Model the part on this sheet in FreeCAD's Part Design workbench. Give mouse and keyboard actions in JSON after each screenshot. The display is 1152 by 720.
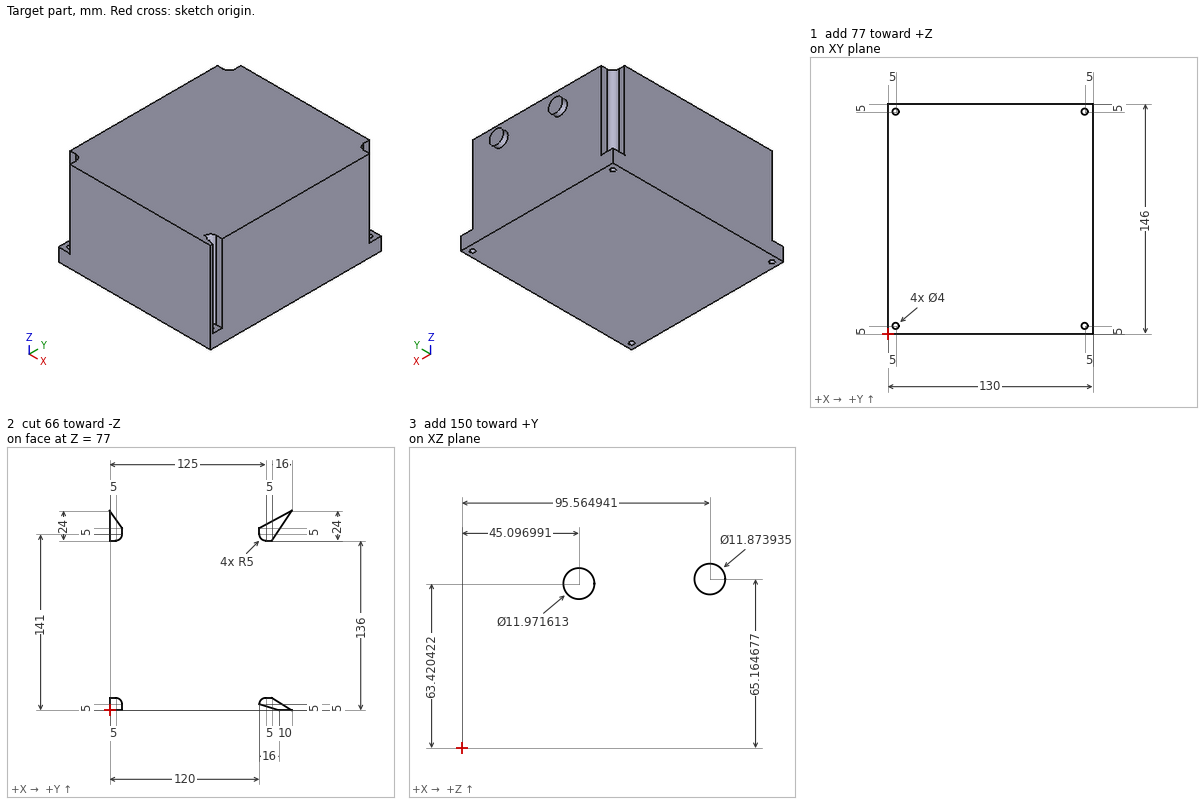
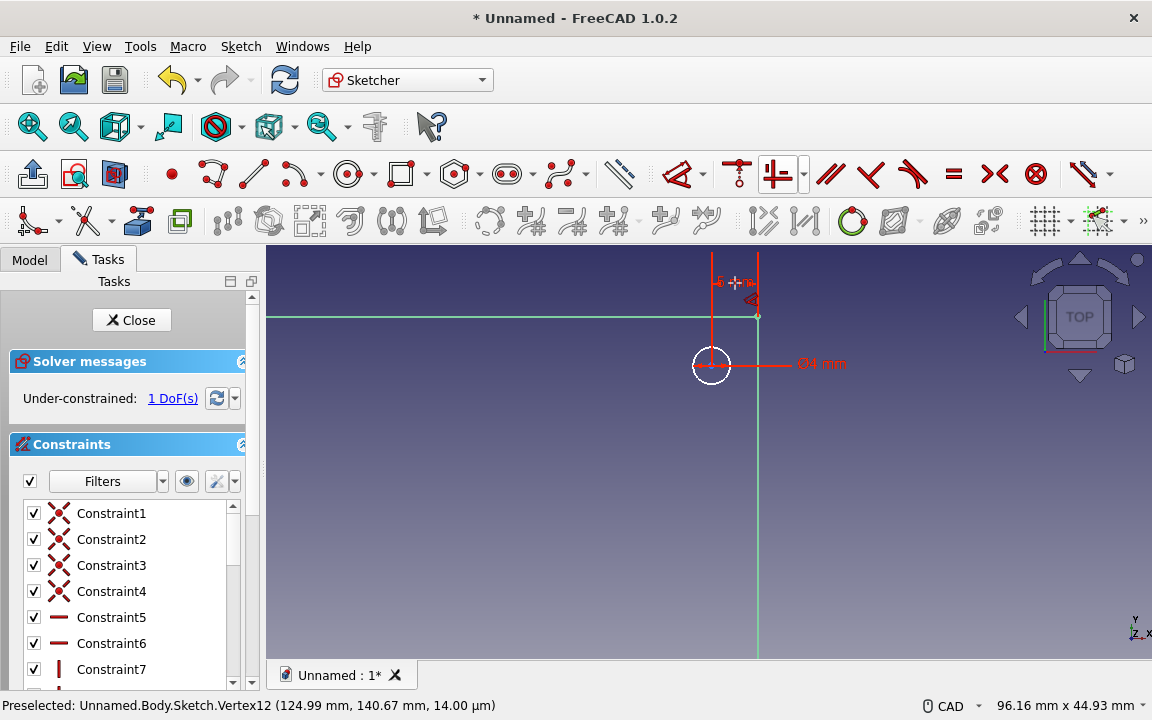
{"action": "left_click", "coordinate": [758, 317]}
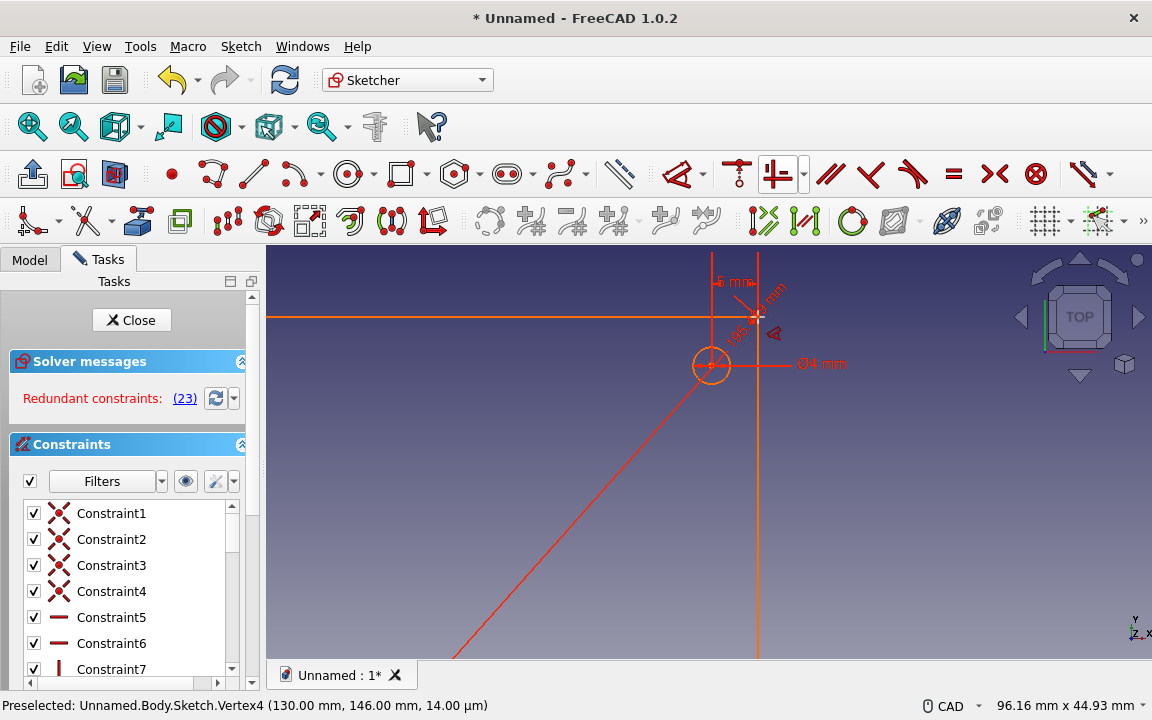
{"action": "left_click", "coordinate": [712, 366]}
{"action": "left_click", "coordinate": [792, 341]}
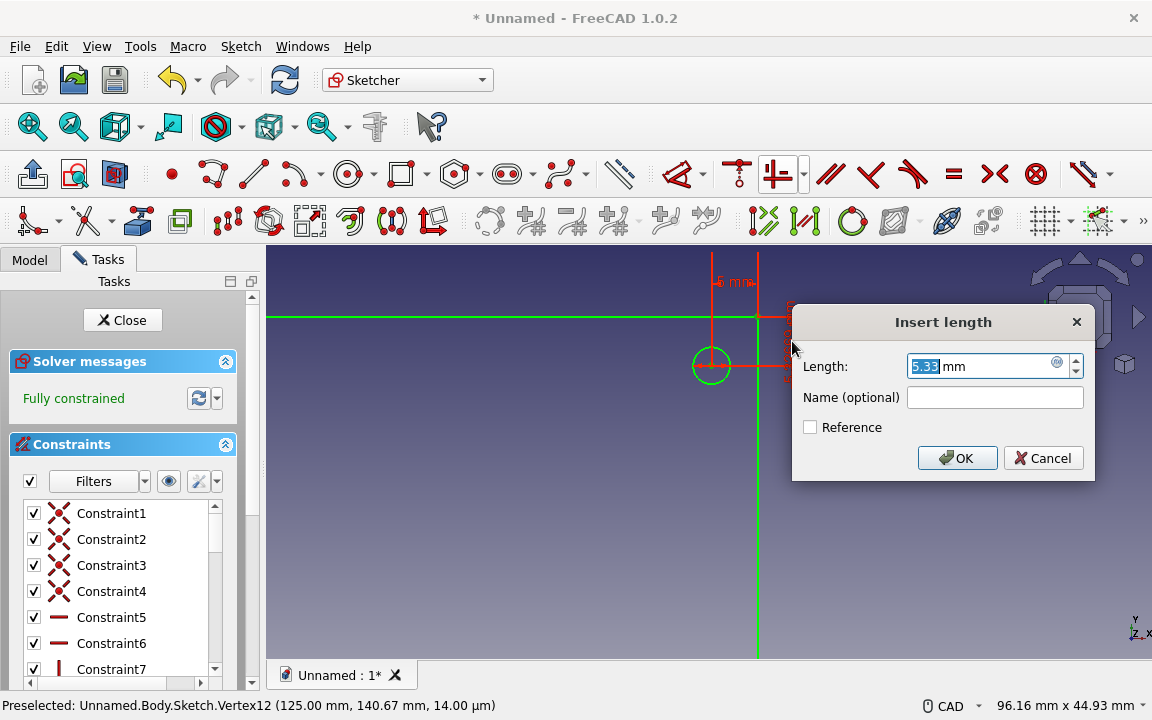
{"action": "type", "text": "5"}
{"action": "key", "text": "Return"}
{"action": "key", "text": "Escape"}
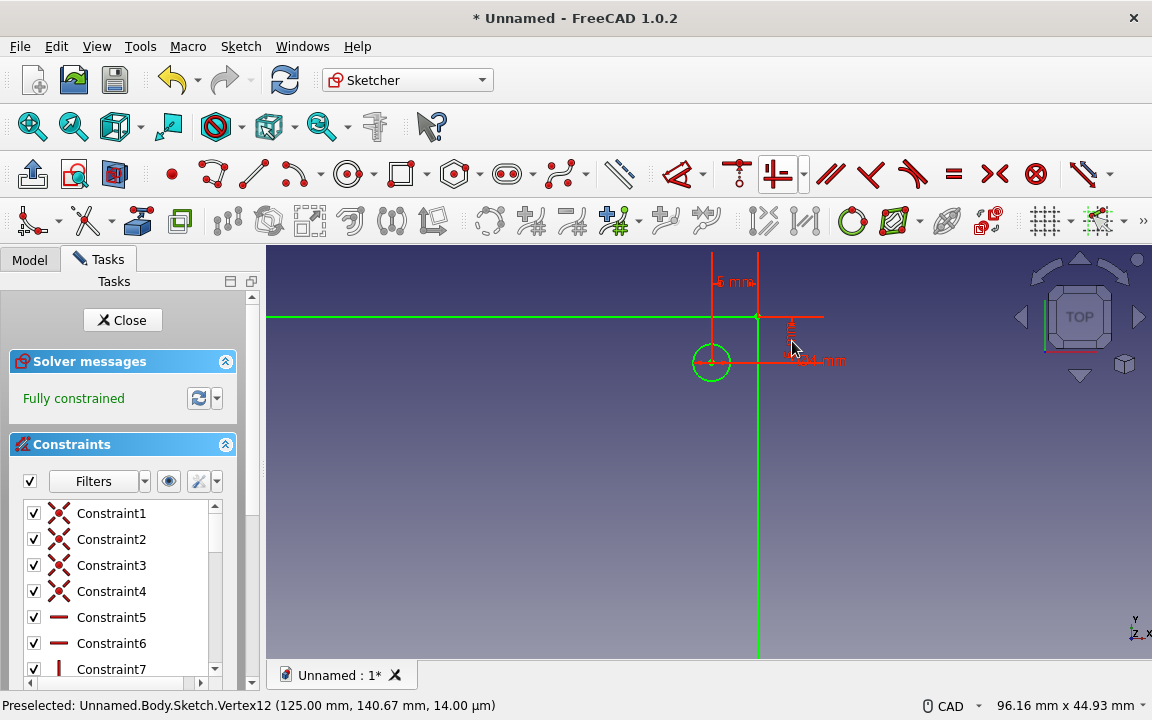
{"action": "left_click", "coordinate": [123, 320]}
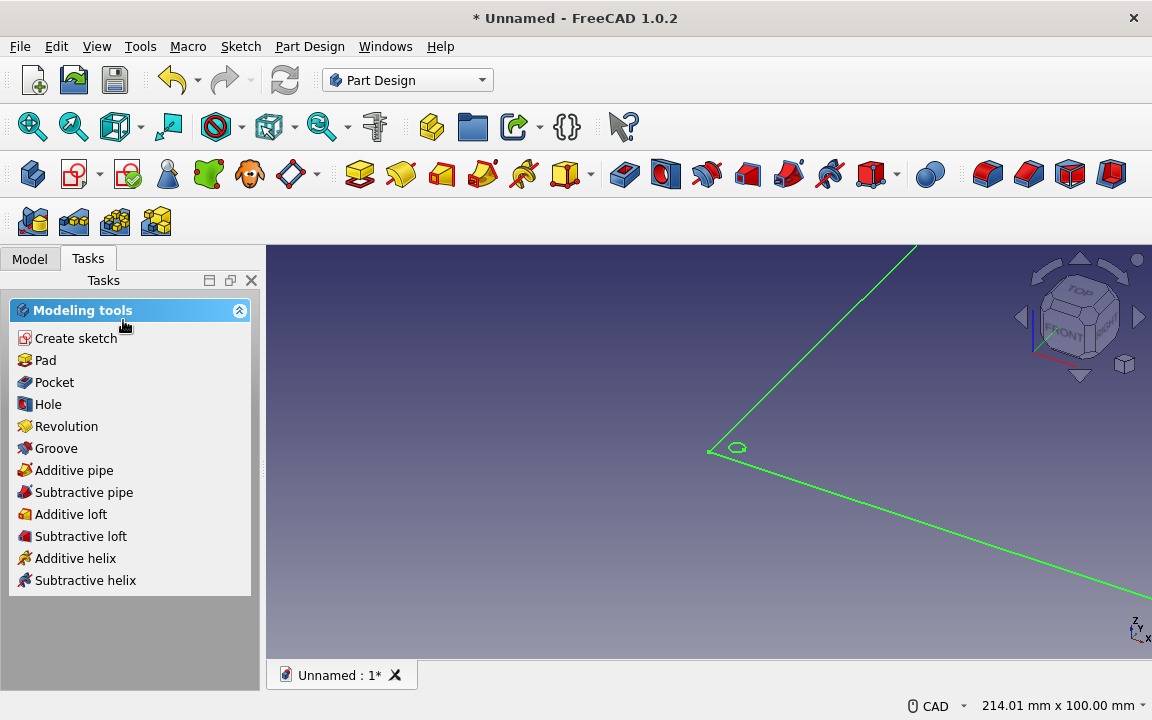
{"action": "left_click", "coordinate": [360, 174]}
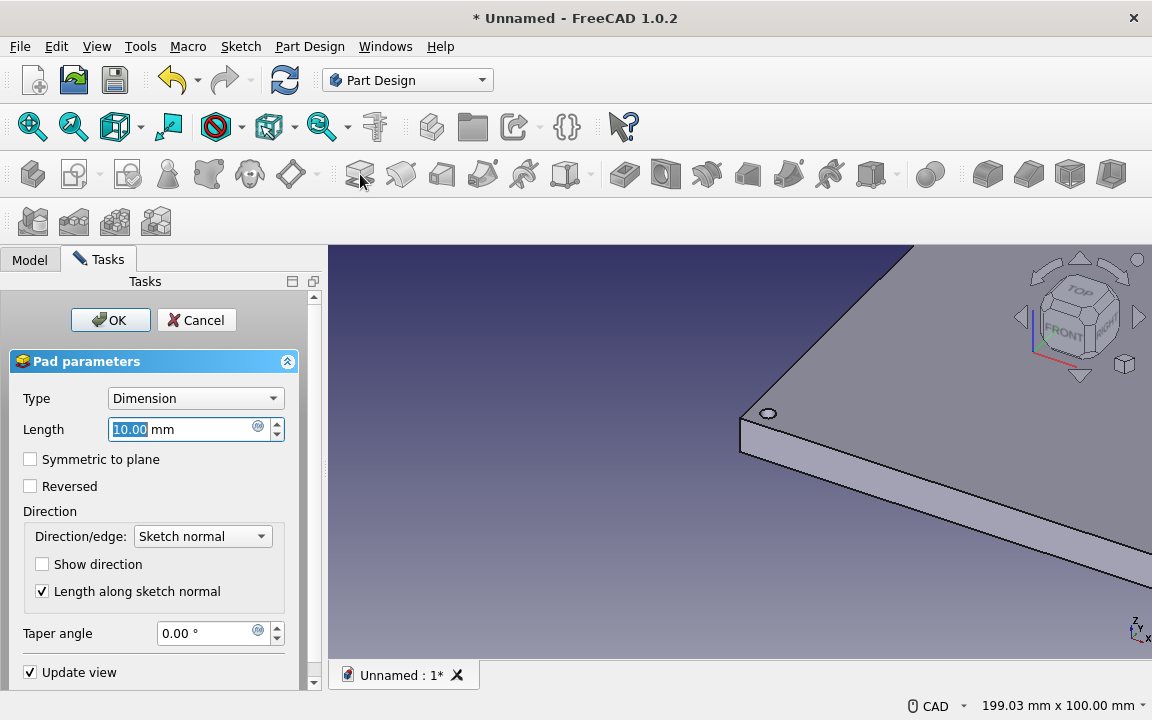
{"action": "type", "text": "77"}
{"action": "key", "text": "Tab"}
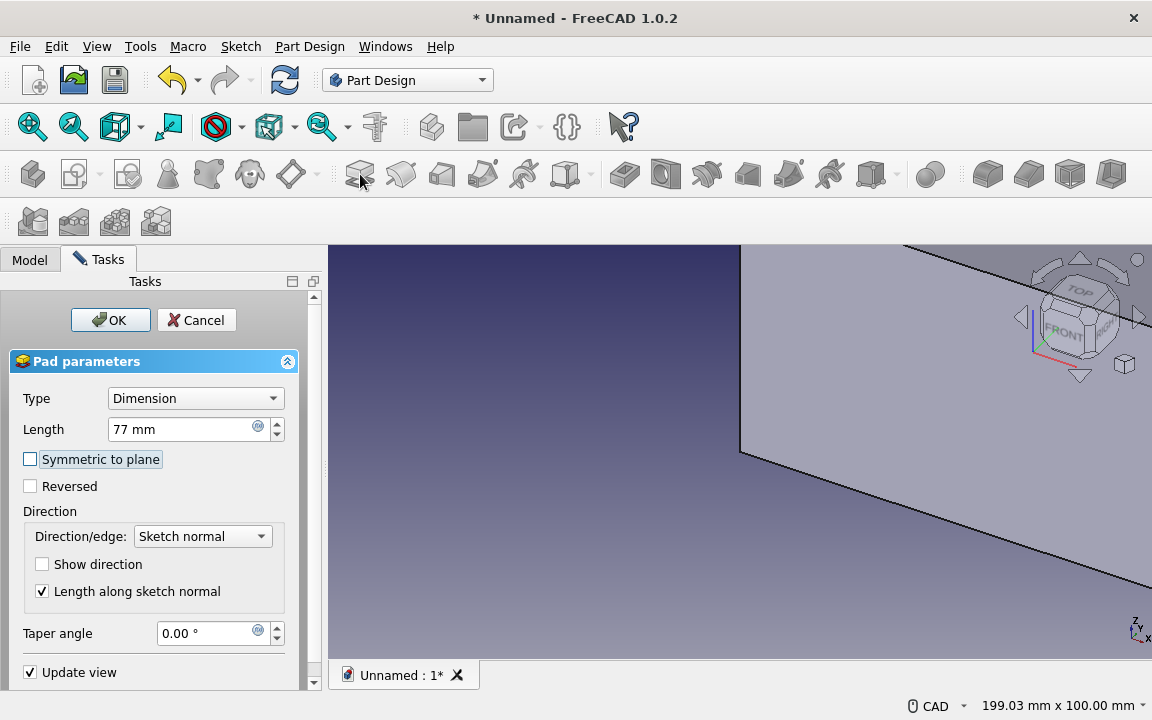
{"action": "left_click", "coordinate": [111, 320]}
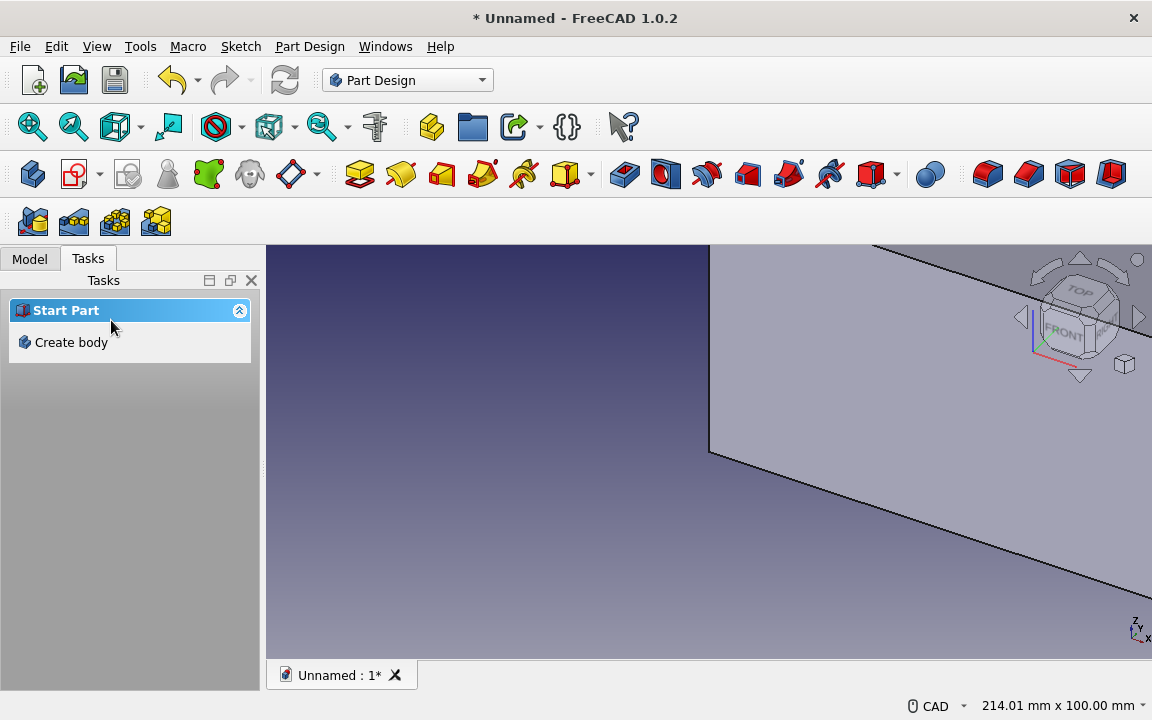
{"action": "left_click", "coordinate": [33, 128]}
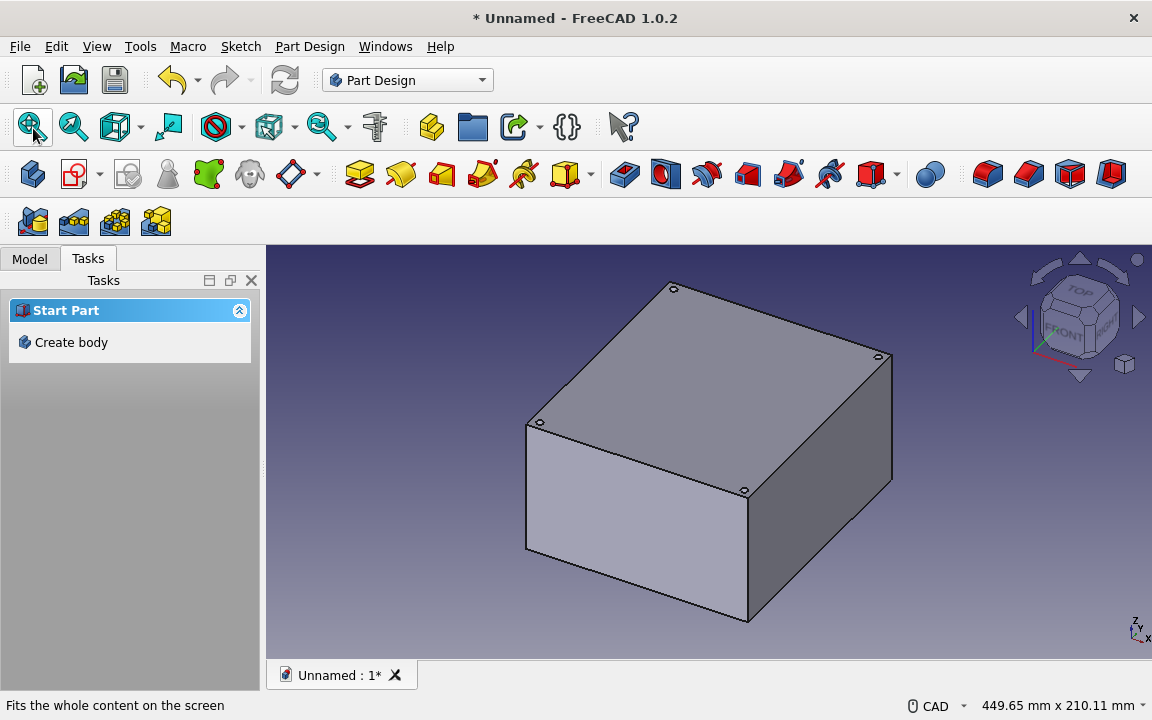
{"action": "left_click", "coordinate": [709, 389]}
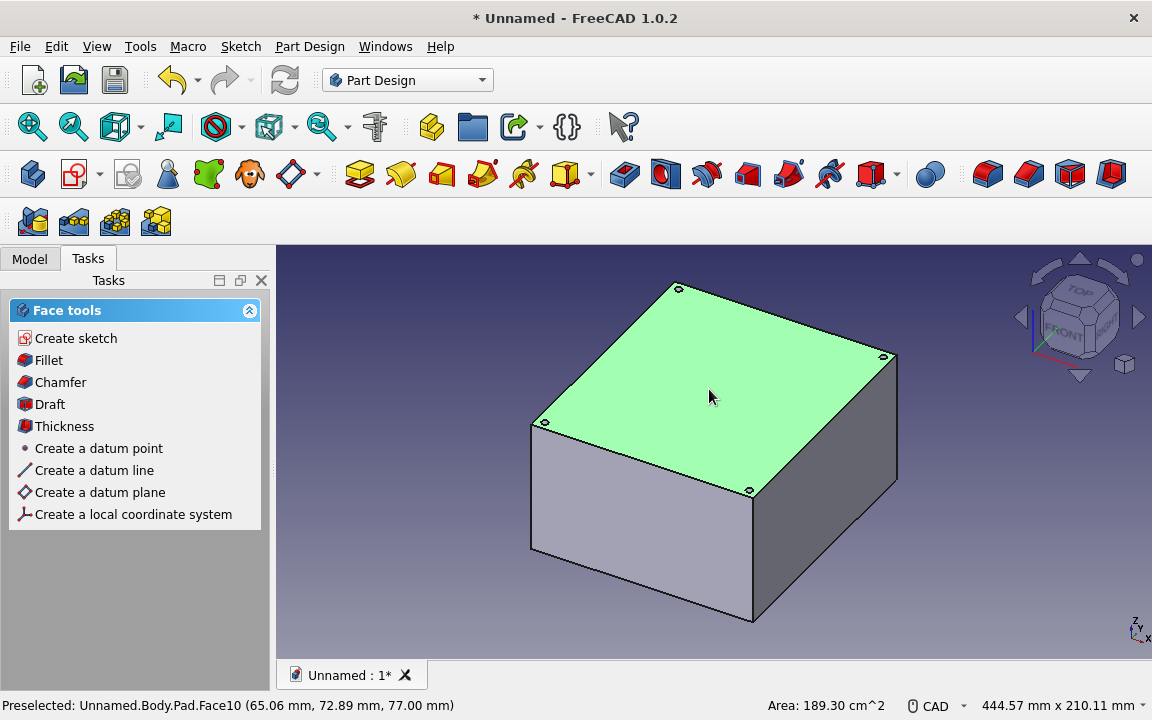
{"action": "left_click", "coordinate": [74, 174]}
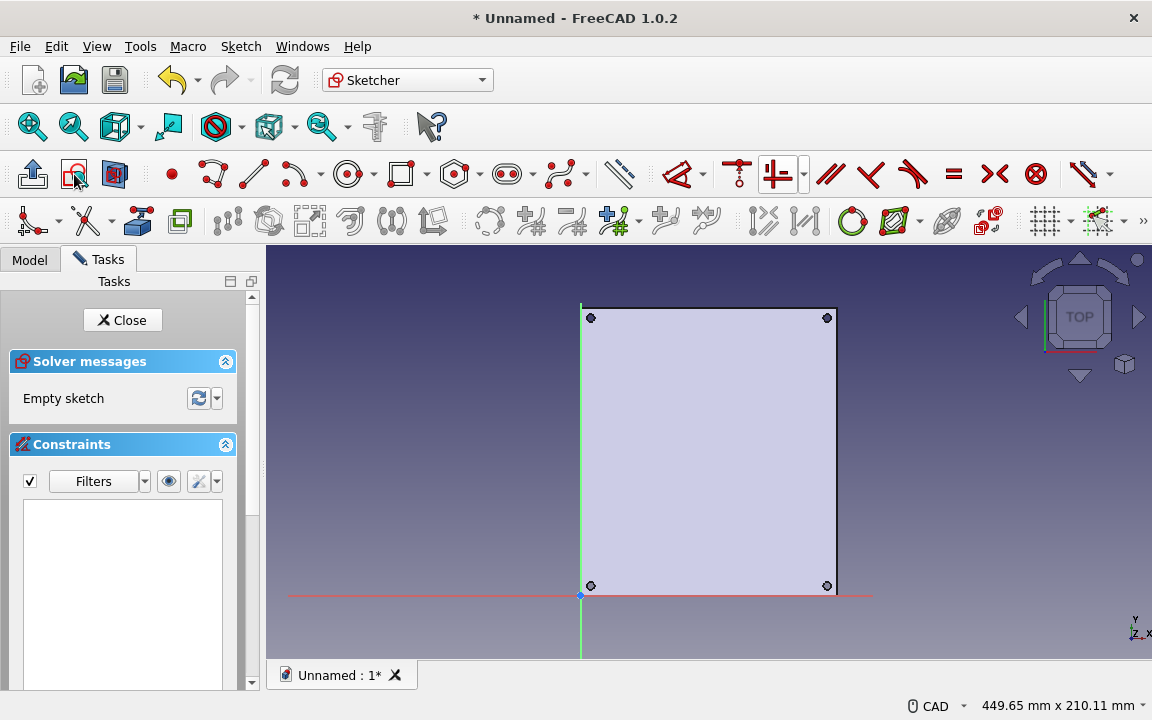
{"action": "scroll", "coordinate": [294, 514], "scroll_direction": "down", "scroll_amount": 1}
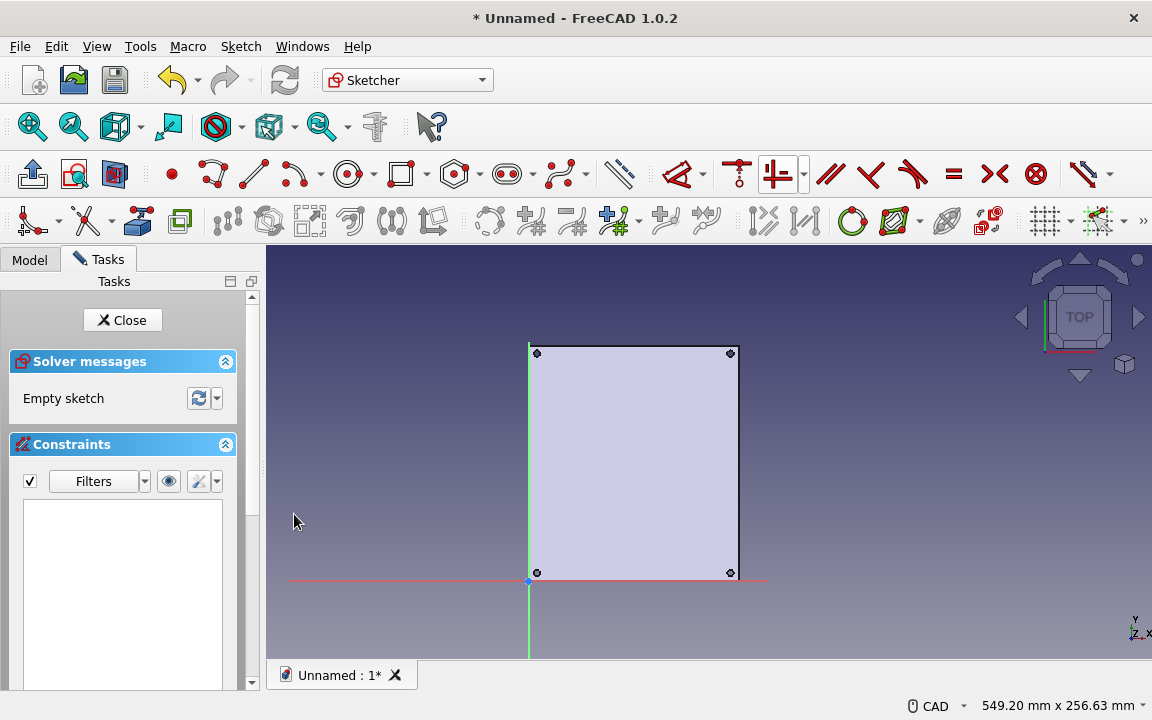
{"action": "left_click", "coordinate": [213, 174]}